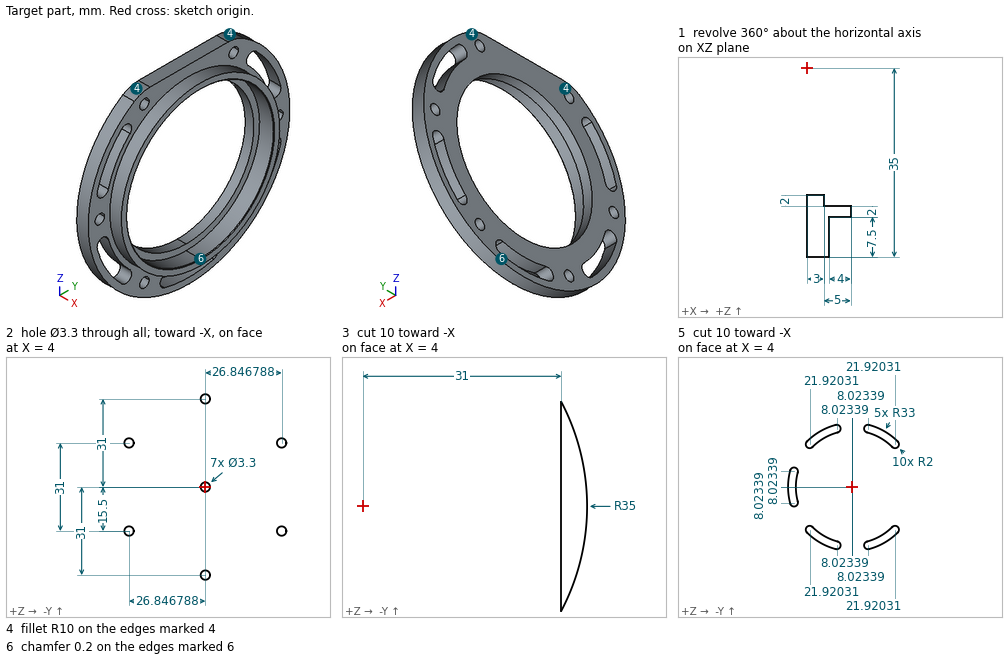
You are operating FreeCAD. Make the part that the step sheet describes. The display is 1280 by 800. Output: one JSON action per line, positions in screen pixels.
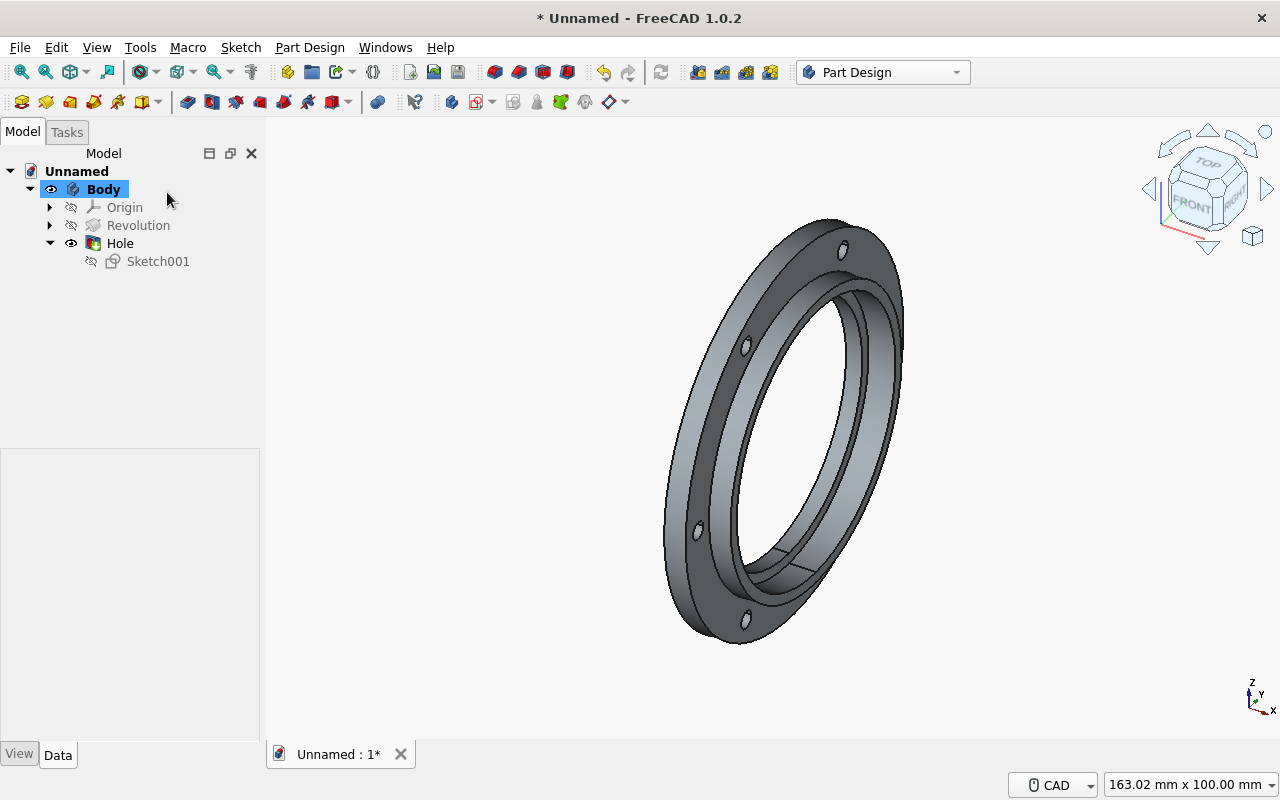
{"action": "left_click", "coordinate": [763, 312]}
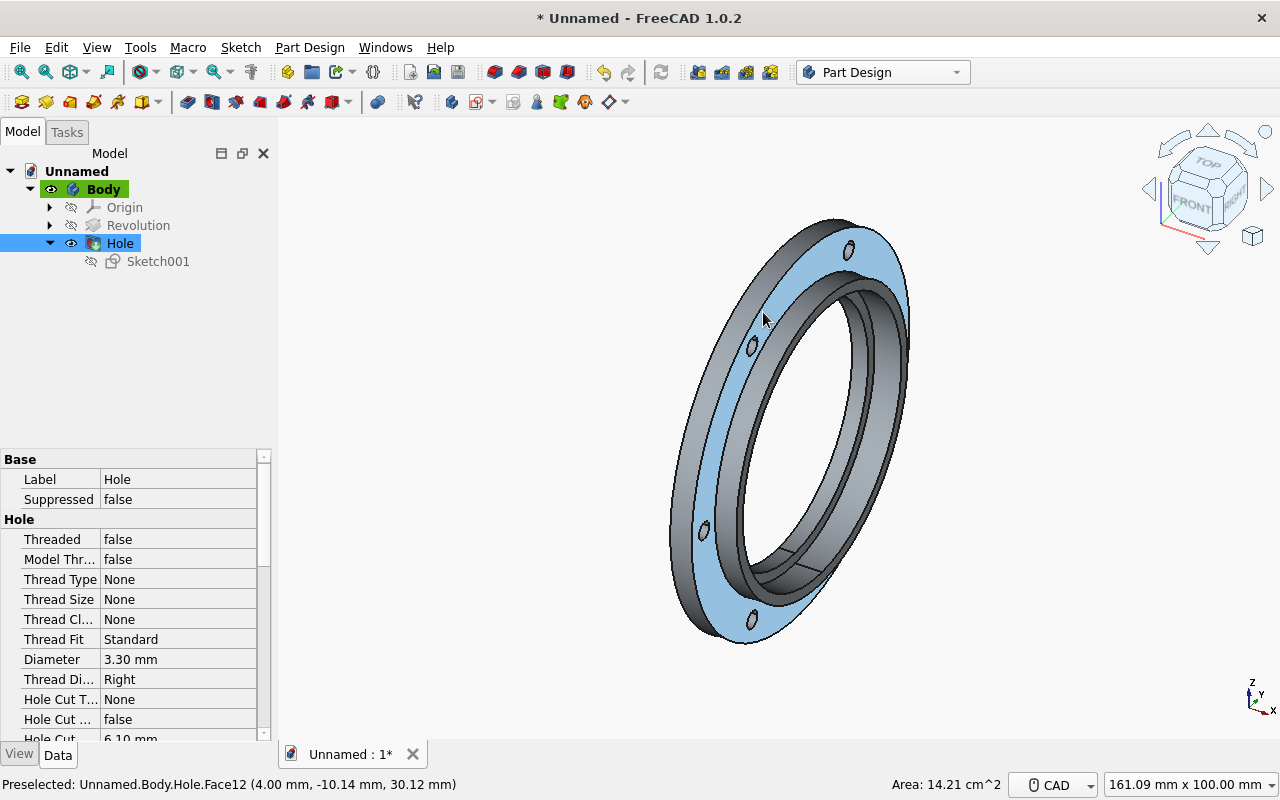
{"action": "left_click", "coordinate": [476, 102]}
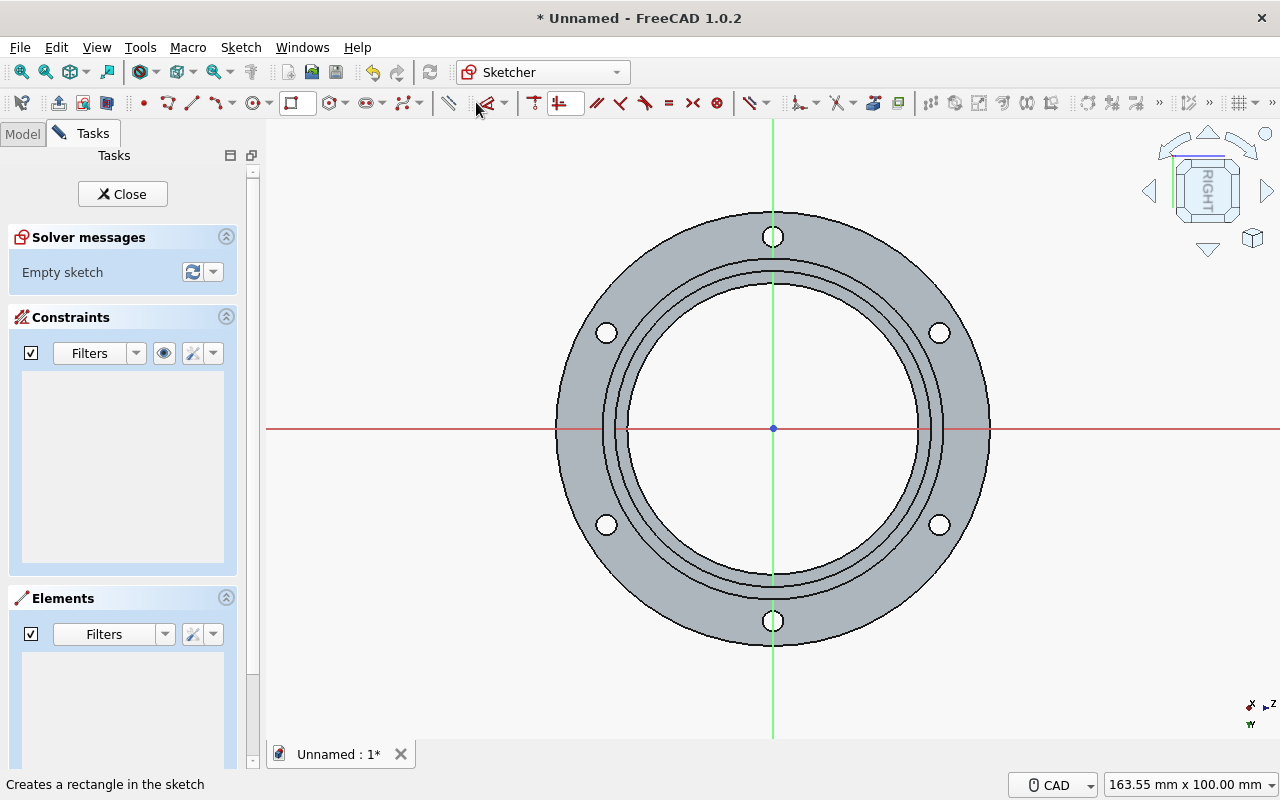
{"action": "left_click", "coordinate": [108, 104]}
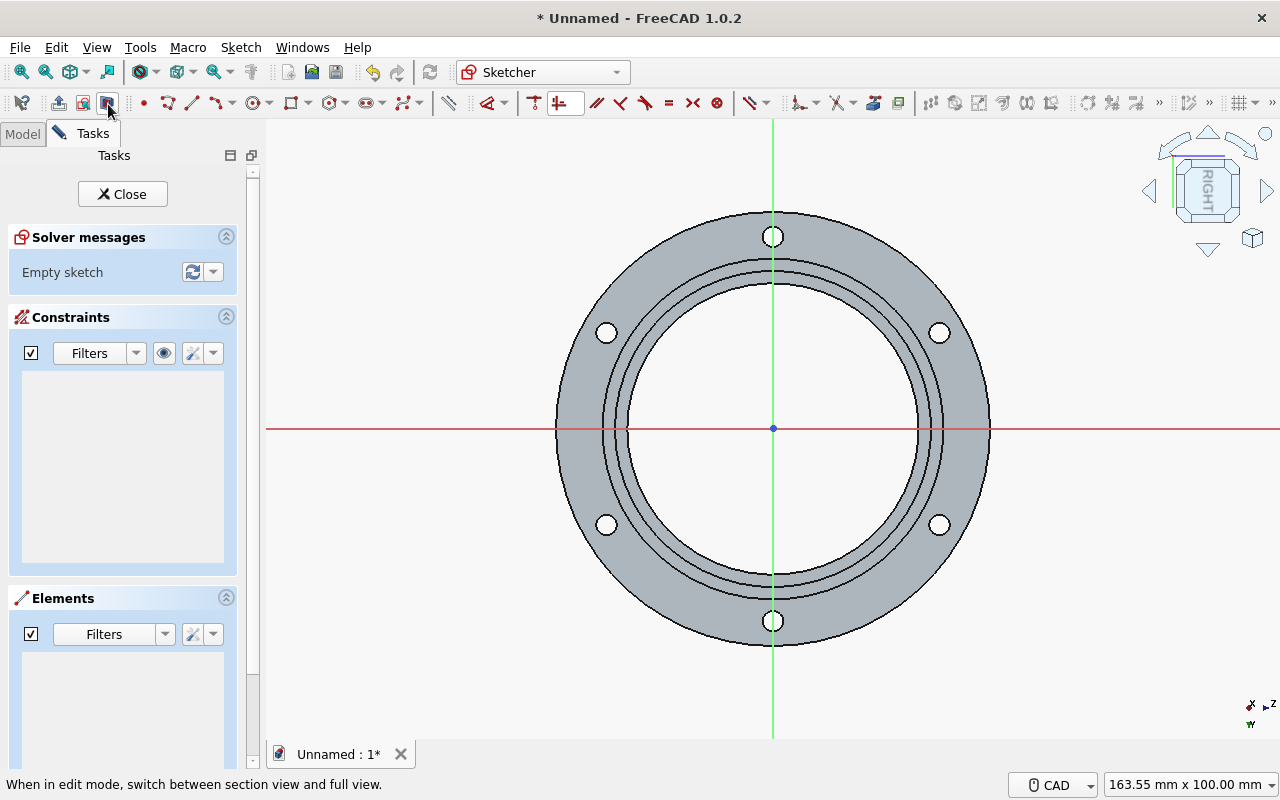
{"action": "scroll", "coordinate": [1097, 429], "scroll_direction": "up", "scroll_amount": 3}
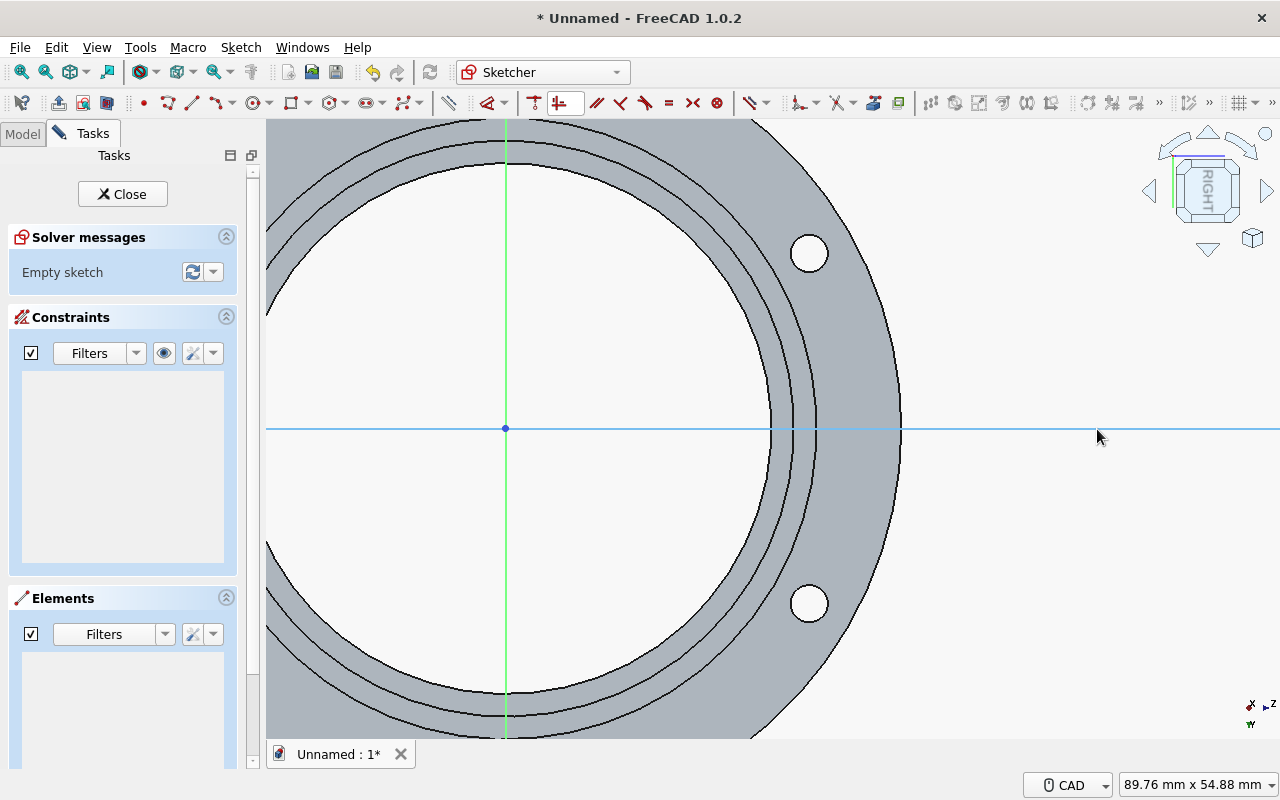
{"action": "left_click", "coordinate": [192, 104]}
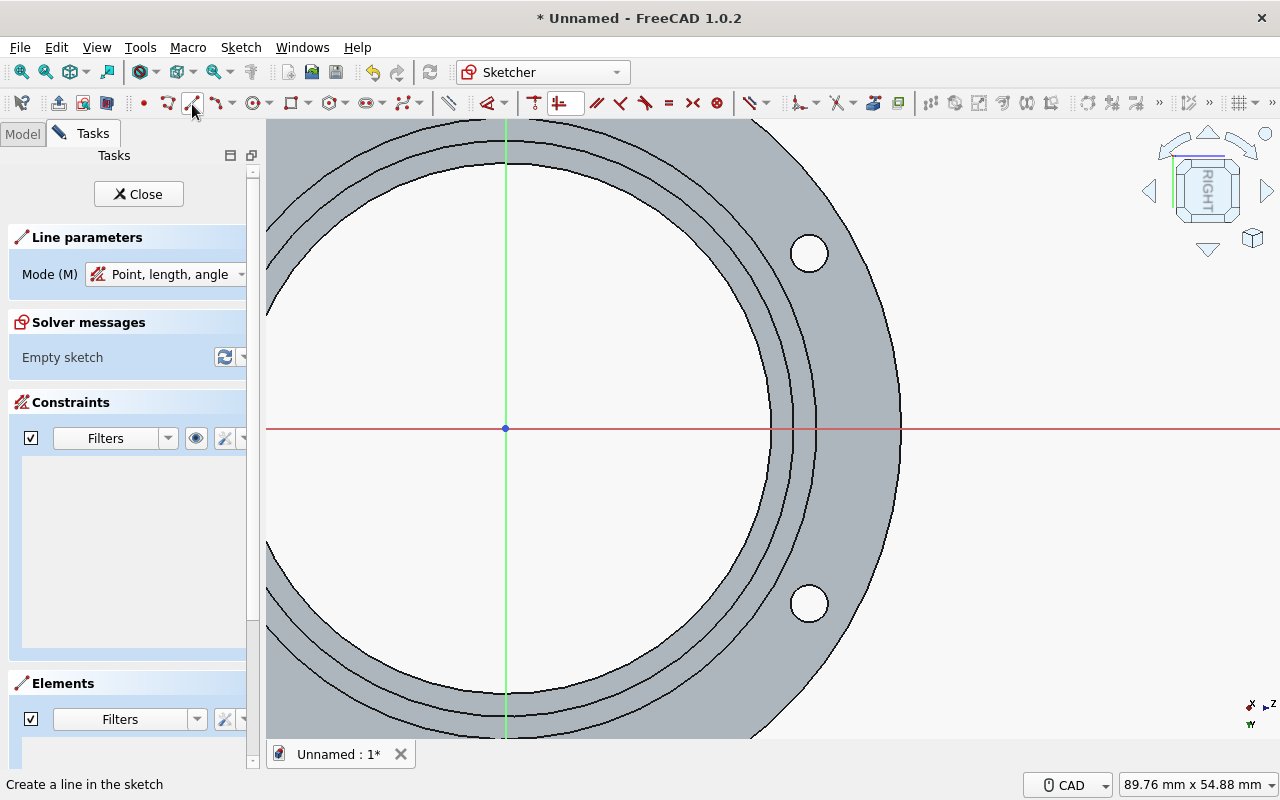
{"action": "left_click", "coordinate": [856, 245]}
{"action": "left_click", "coordinate": [856, 612]}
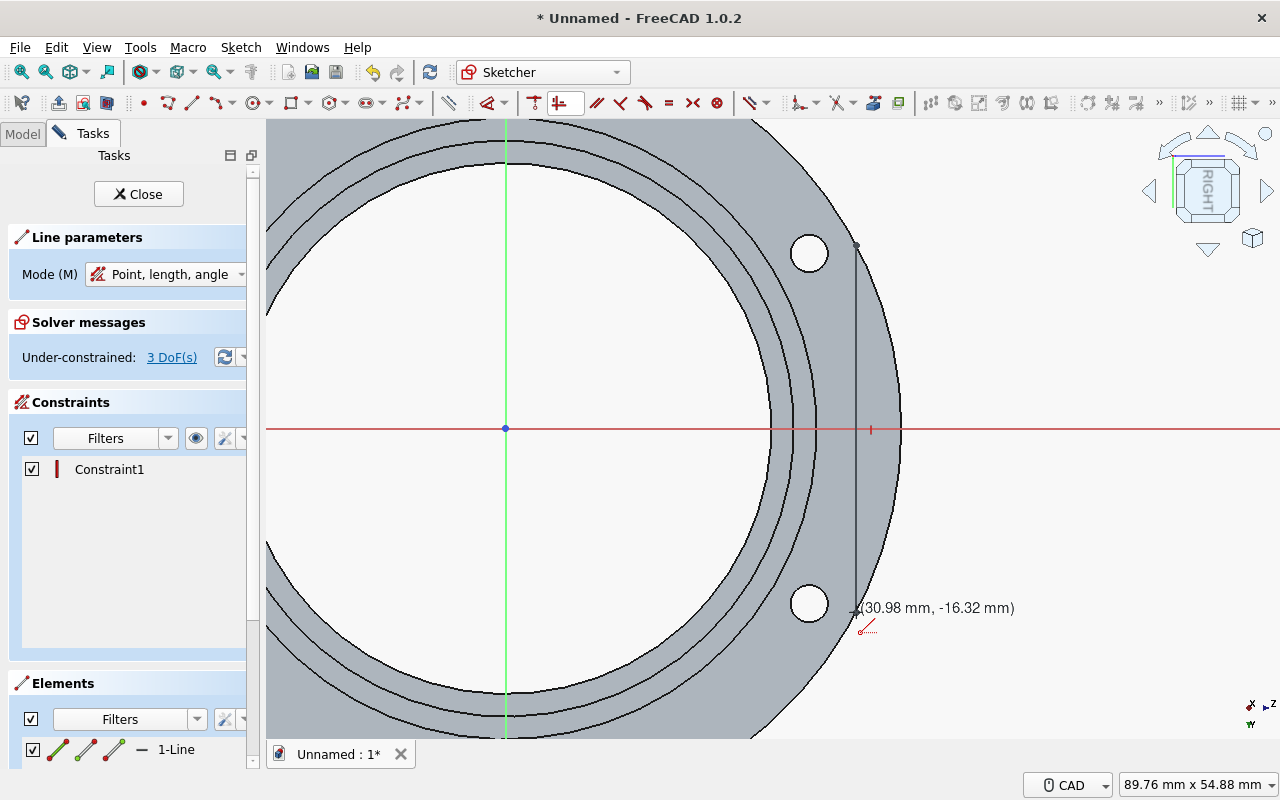
{"action": "left_click", "coordinate": [216, 104]}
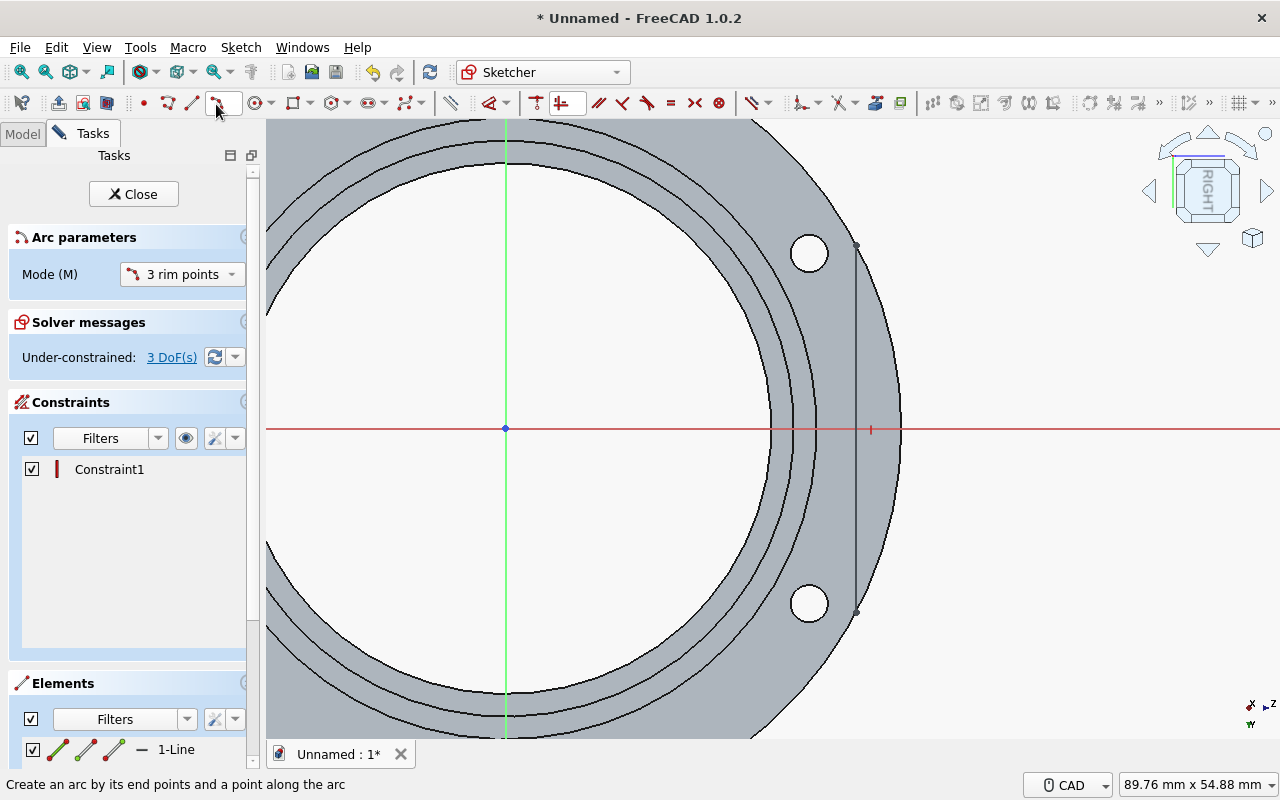
{"action": "left_click", "coordinate": [856, 613]}
{"action": "left_click", "coordinate": [856, 246]}
{"action": "left_click", "coordinate": [900, 467]}
{"action": "key", "text": "Escape"}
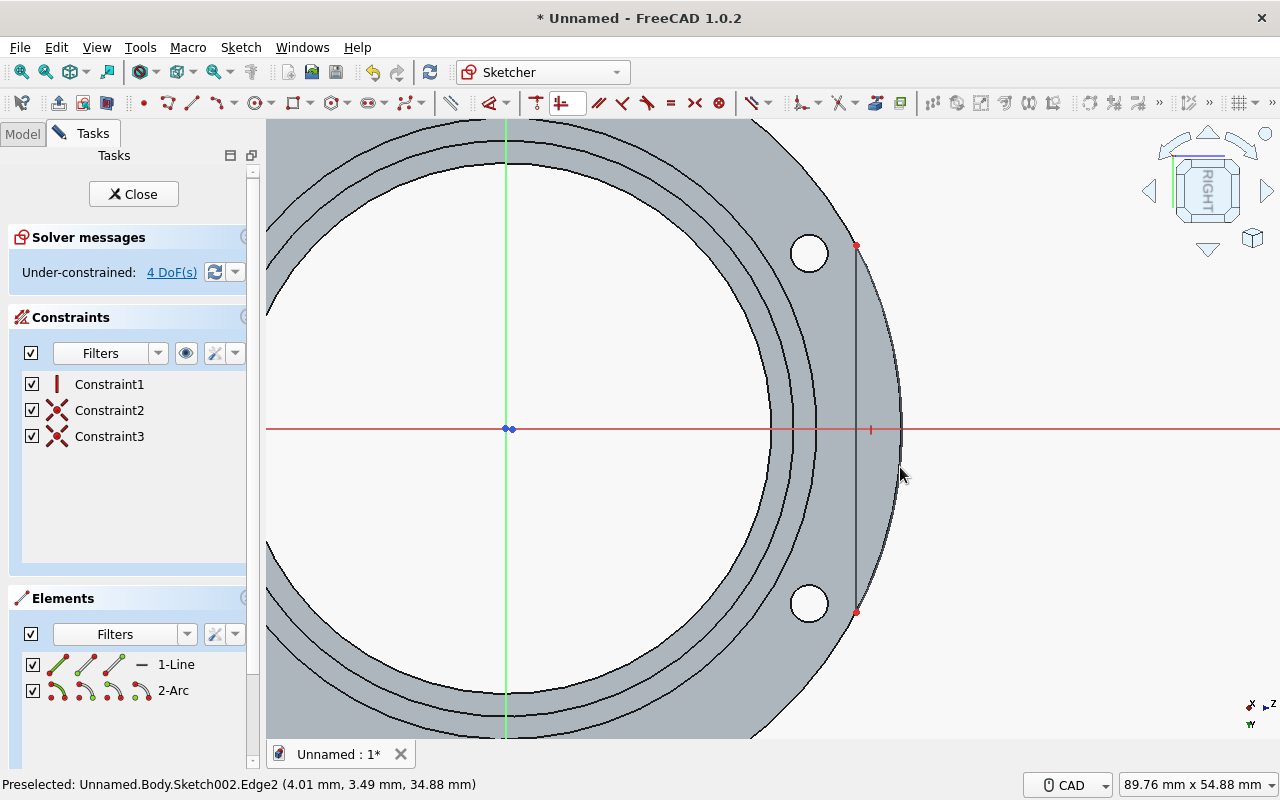
{"action": "left_click_drag", "start_coordinate": [496, 419], "coordinate": [522, 439]}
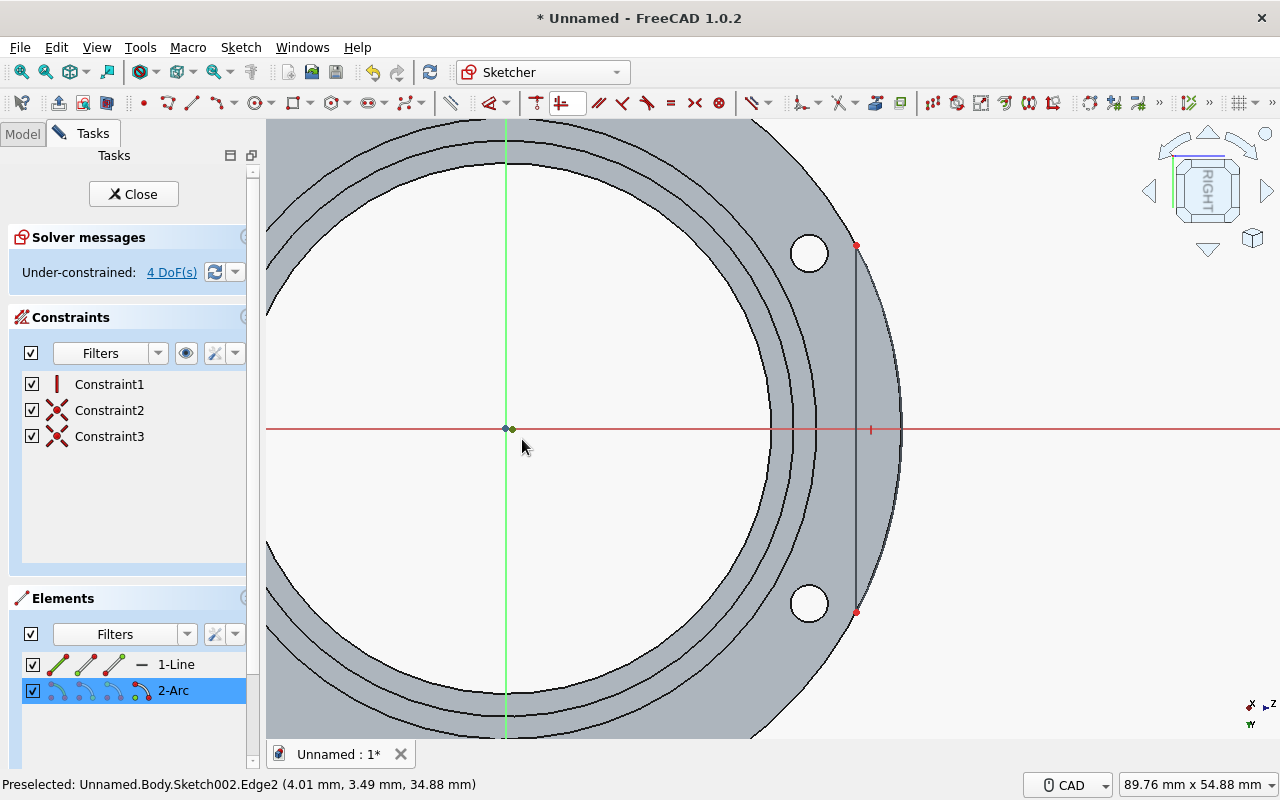
{"action": "left_click", "coordinate": [536, 104]}